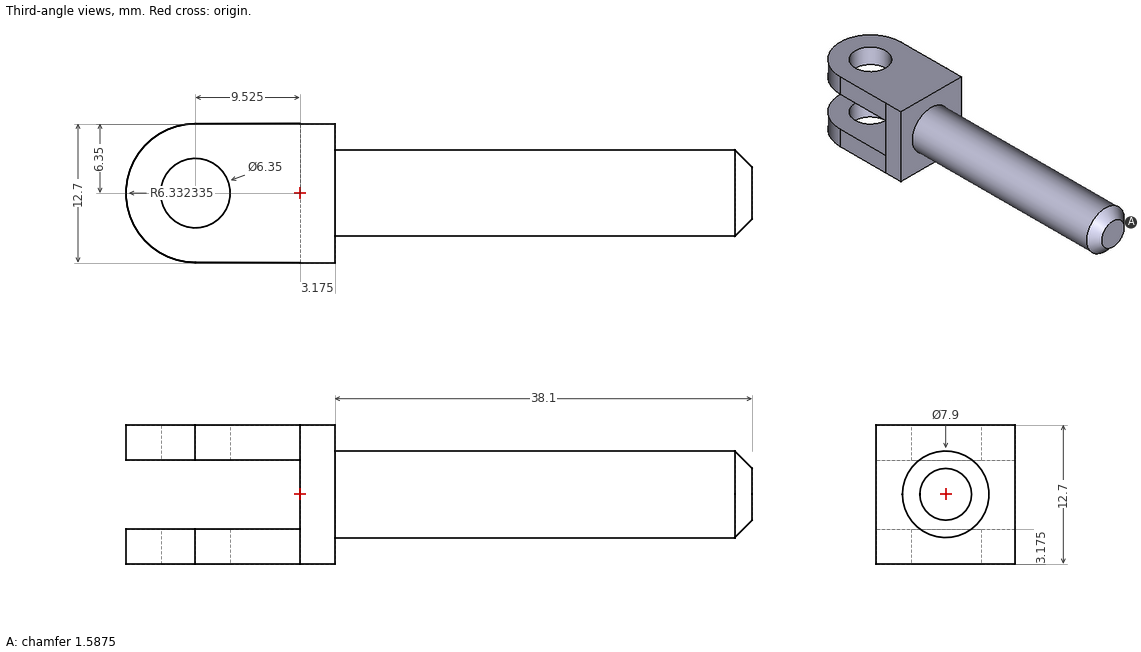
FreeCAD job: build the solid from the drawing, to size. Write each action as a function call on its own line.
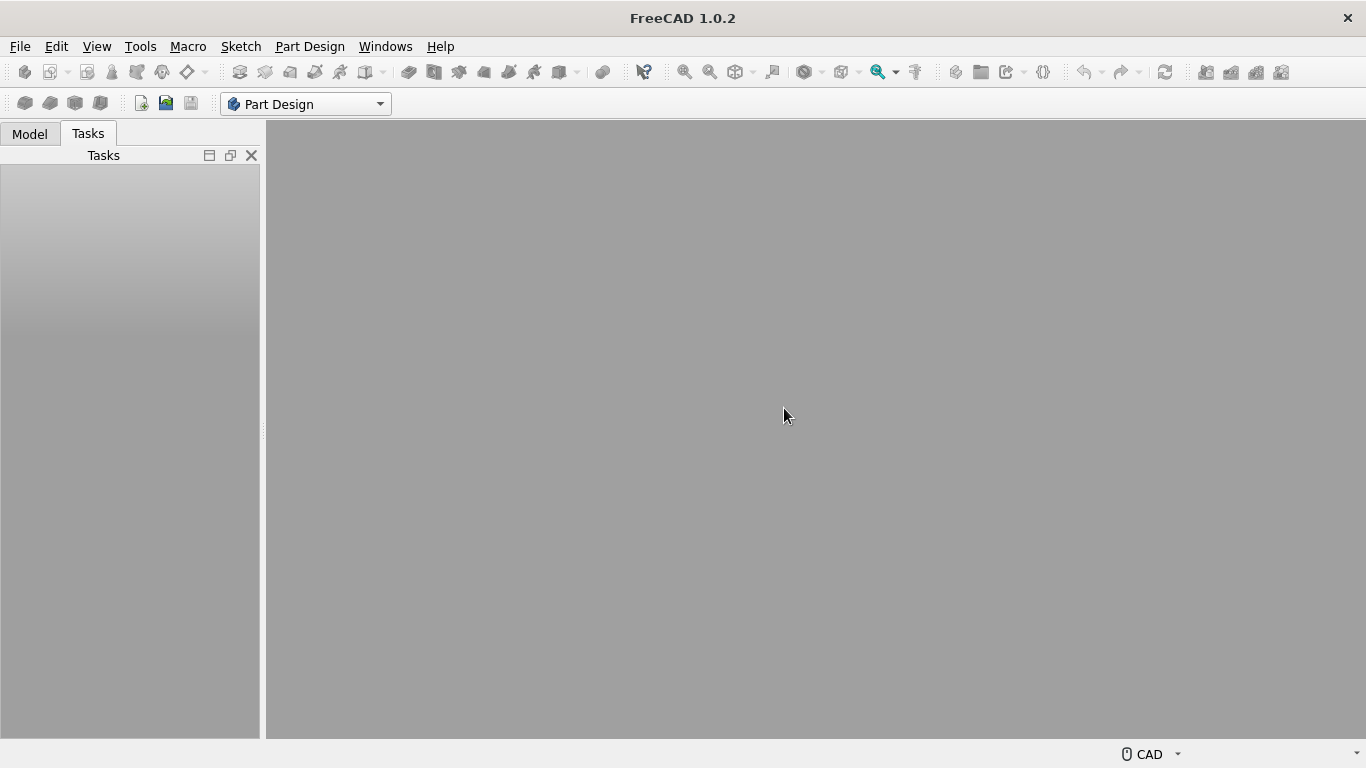
click(141, 104)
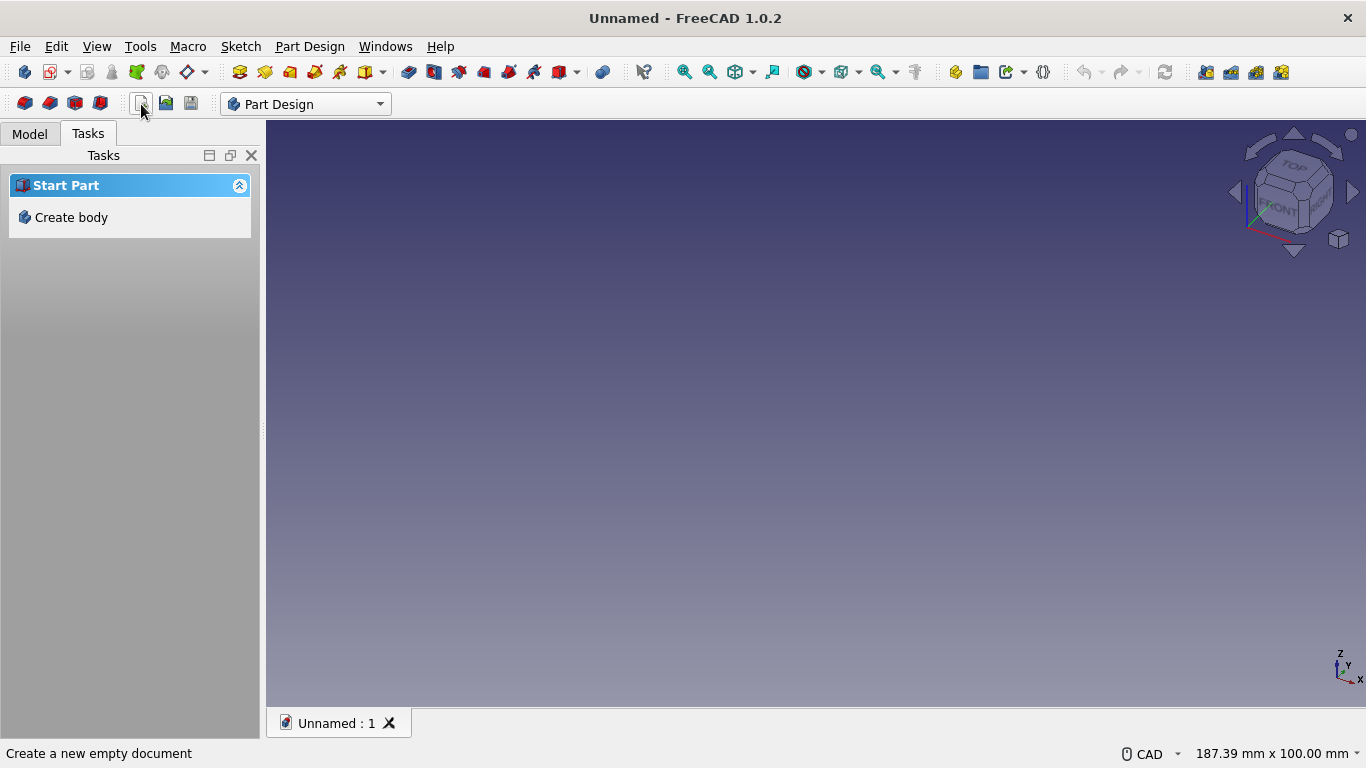
click(50, 72)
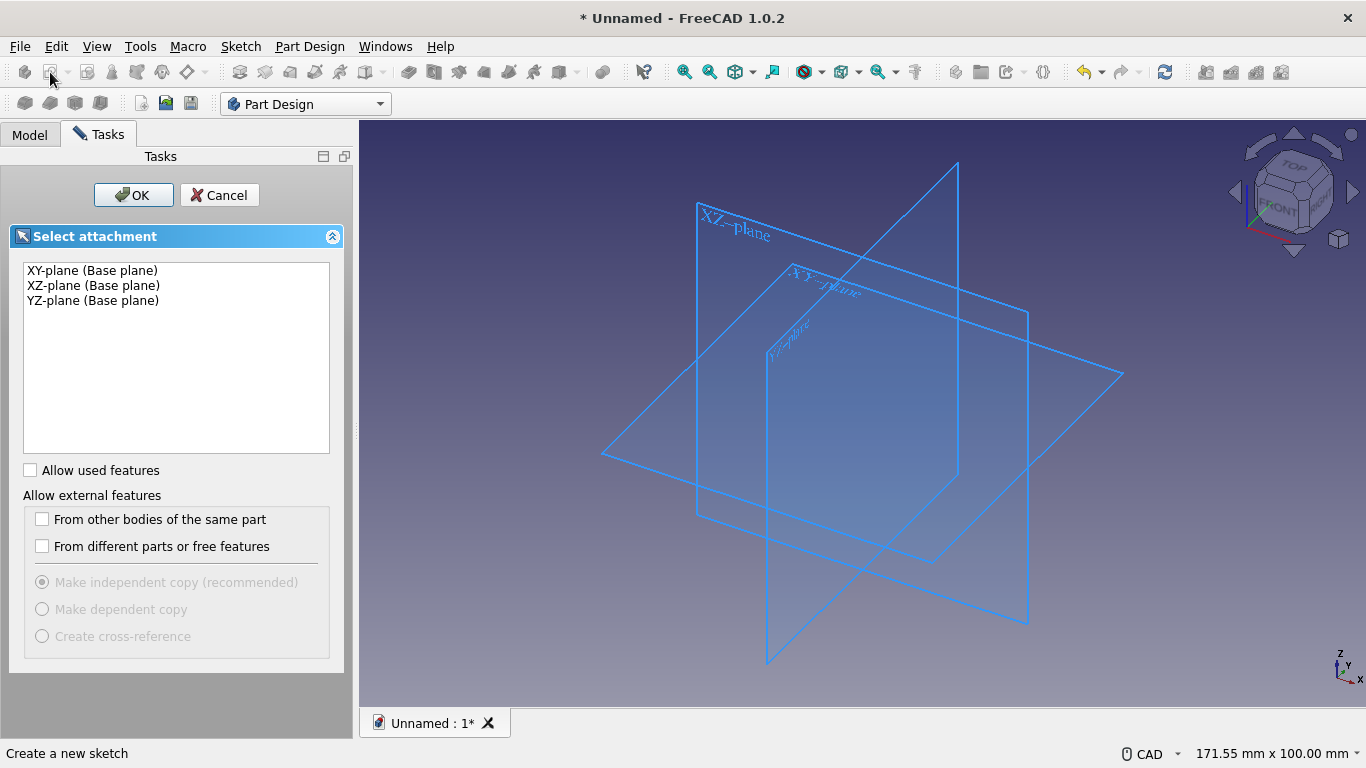
click(84, 270)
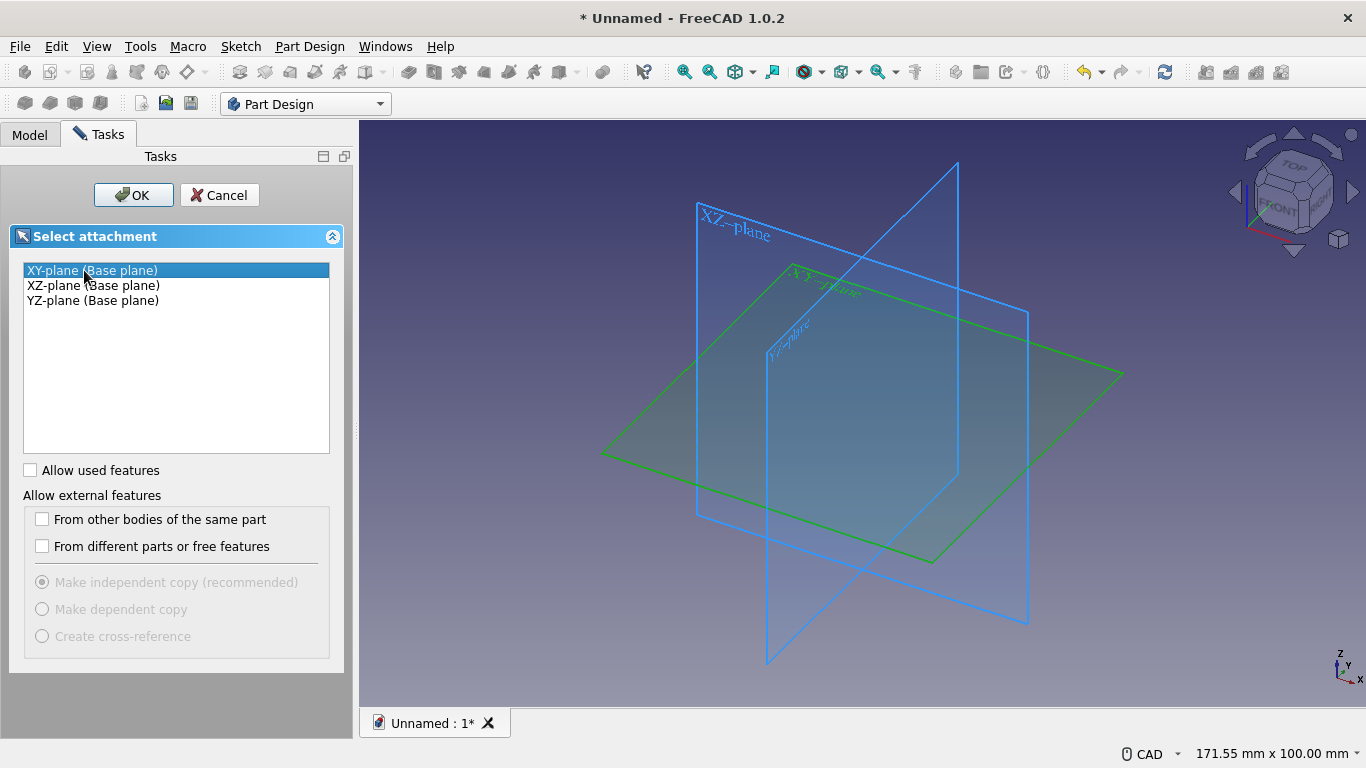
click(134, 195)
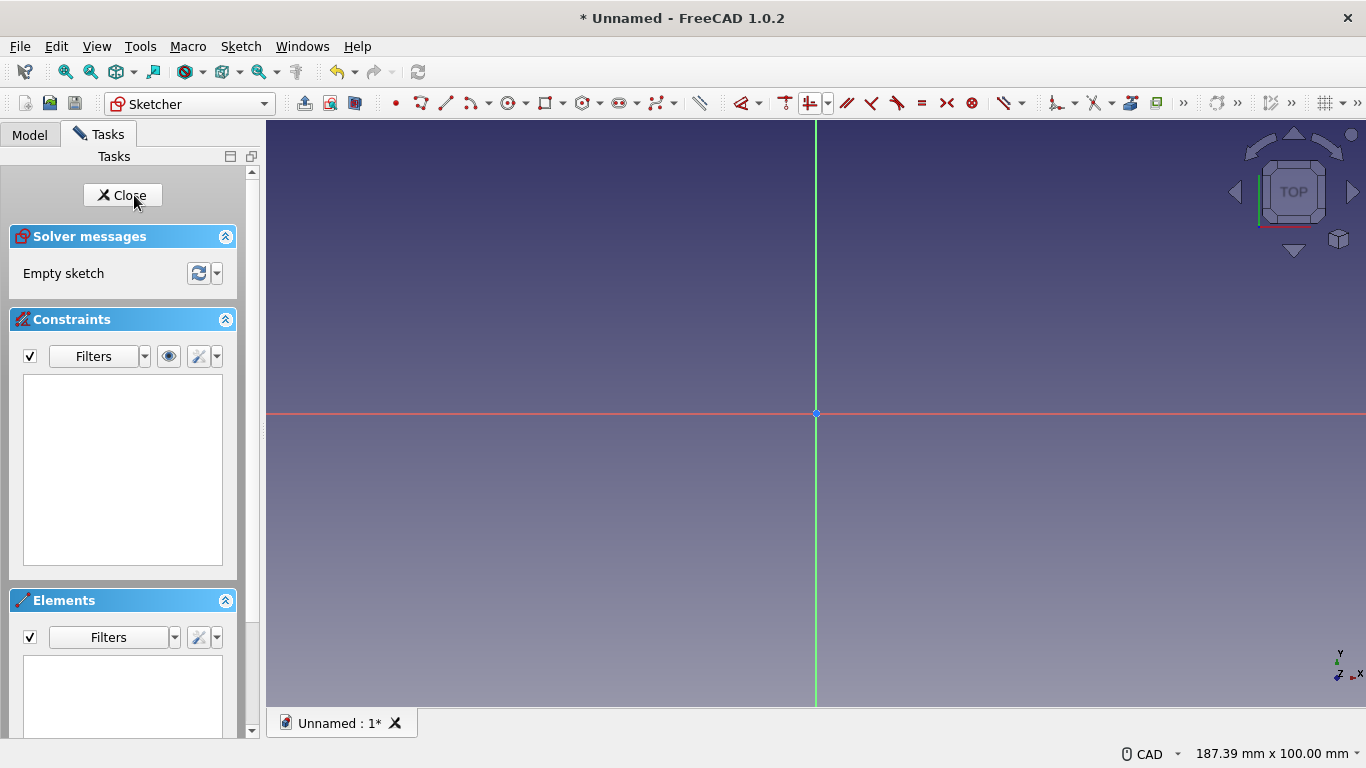
scroll(845, 414, up, 8)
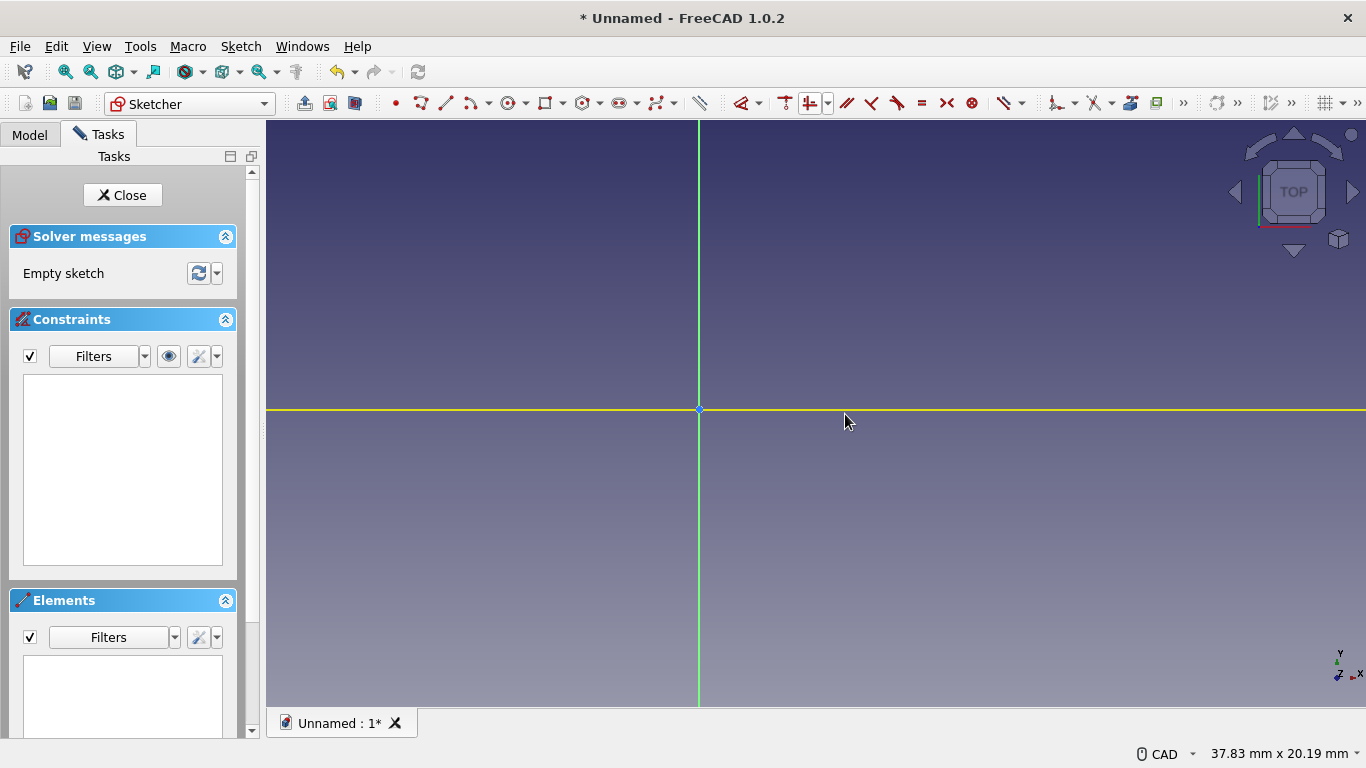
click(544, 104)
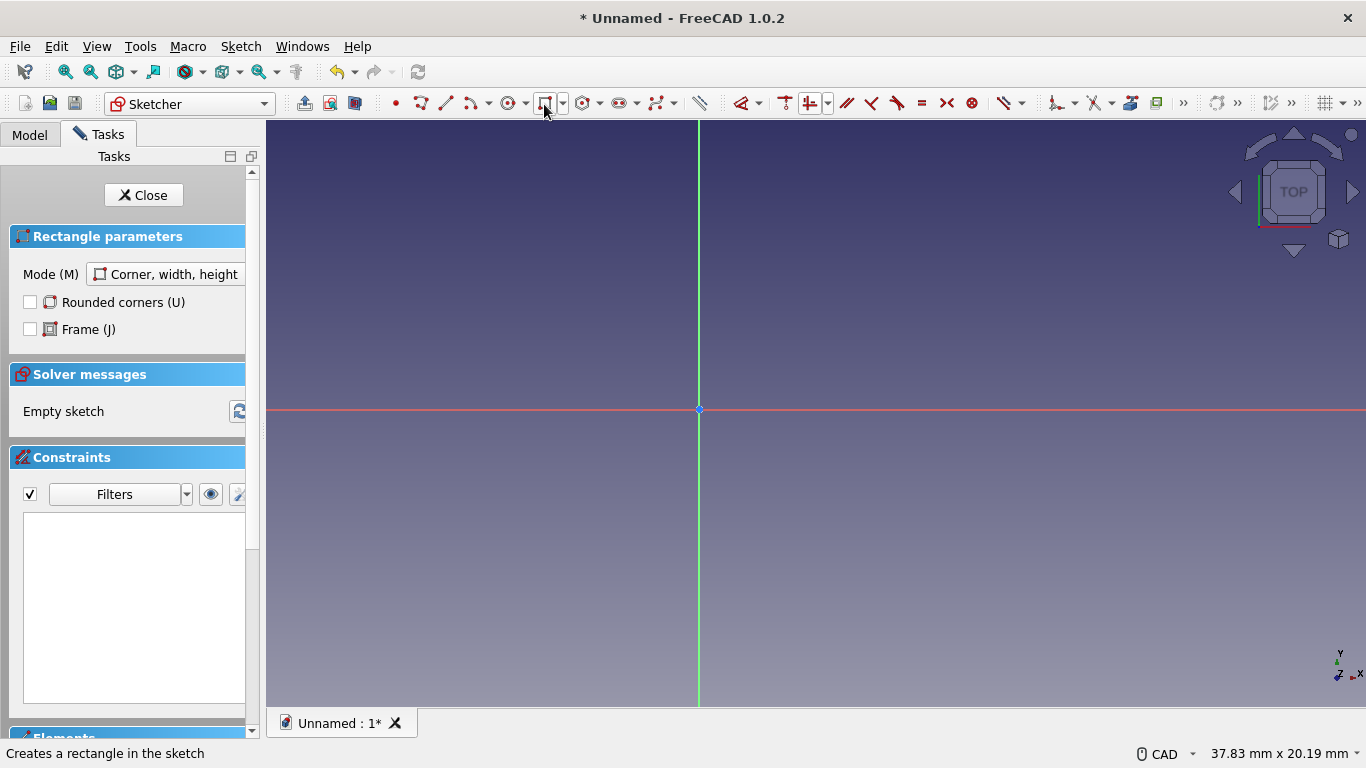
click(699, 225)
move(792, 594)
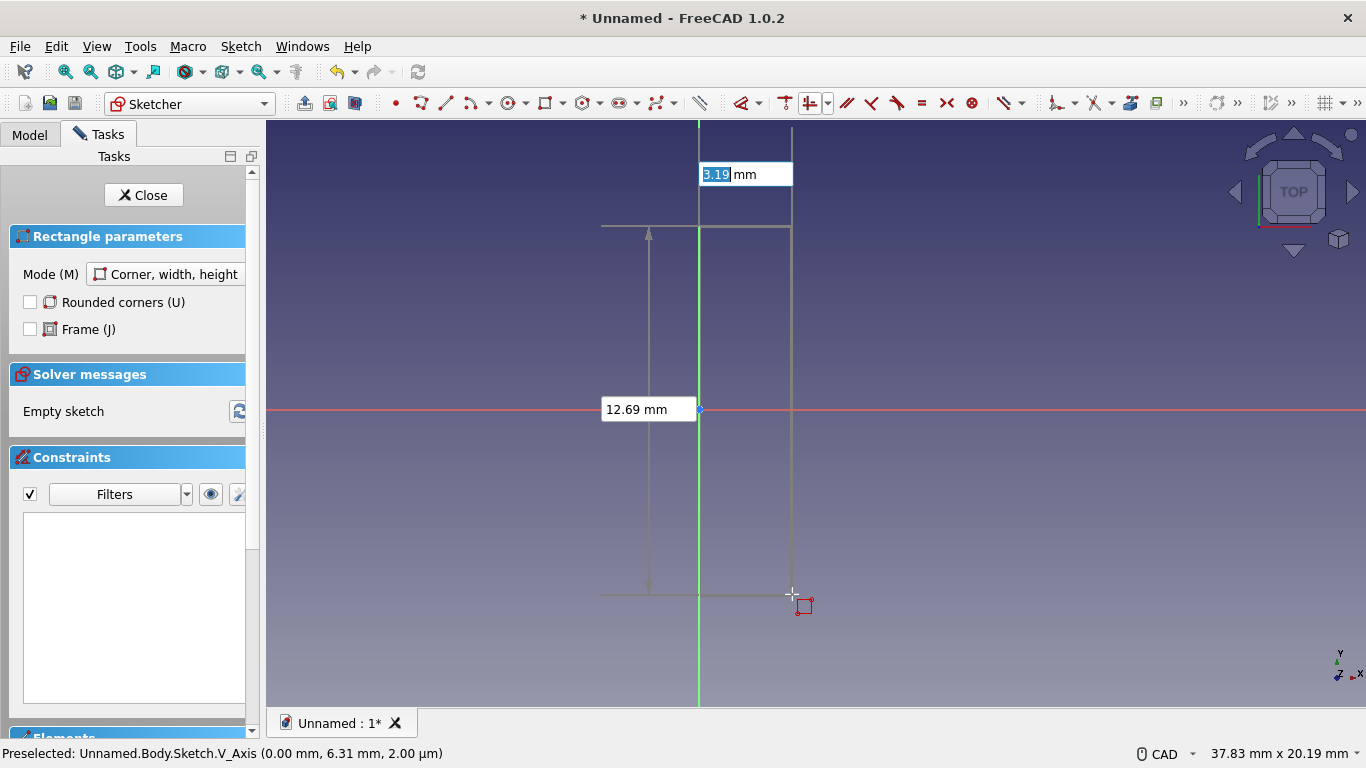
text(3.175)
key(Tab)
text(12.7)
key(Return)
key(Escape)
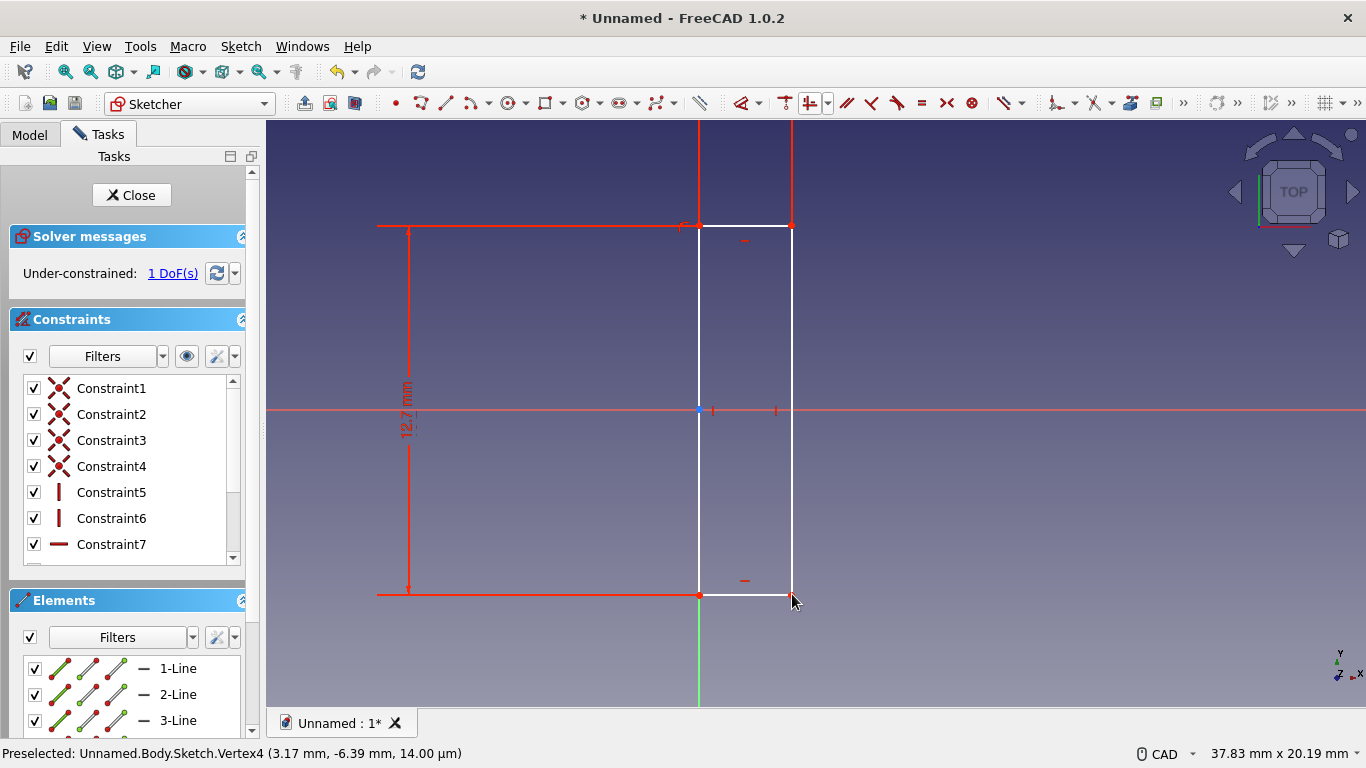
click(740, 104)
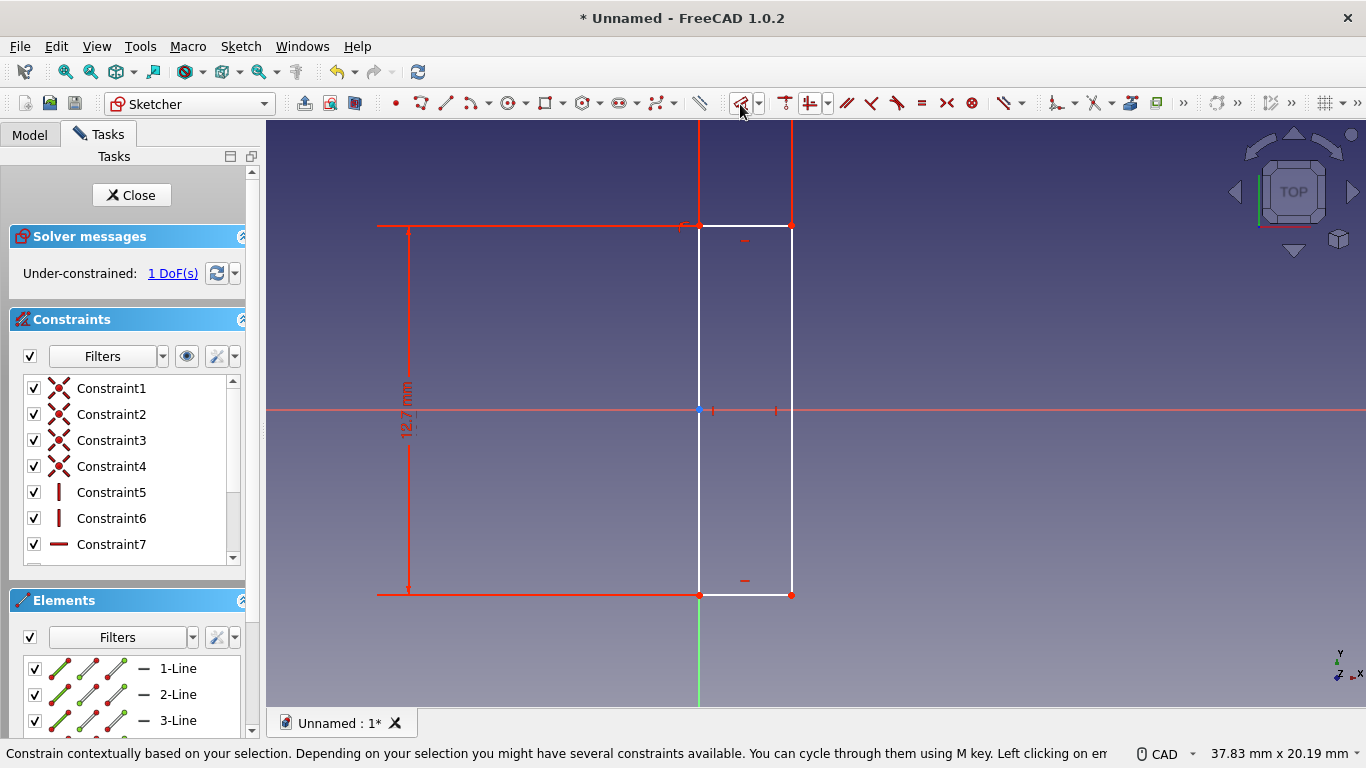
click(699, 226)
click(665, 318)